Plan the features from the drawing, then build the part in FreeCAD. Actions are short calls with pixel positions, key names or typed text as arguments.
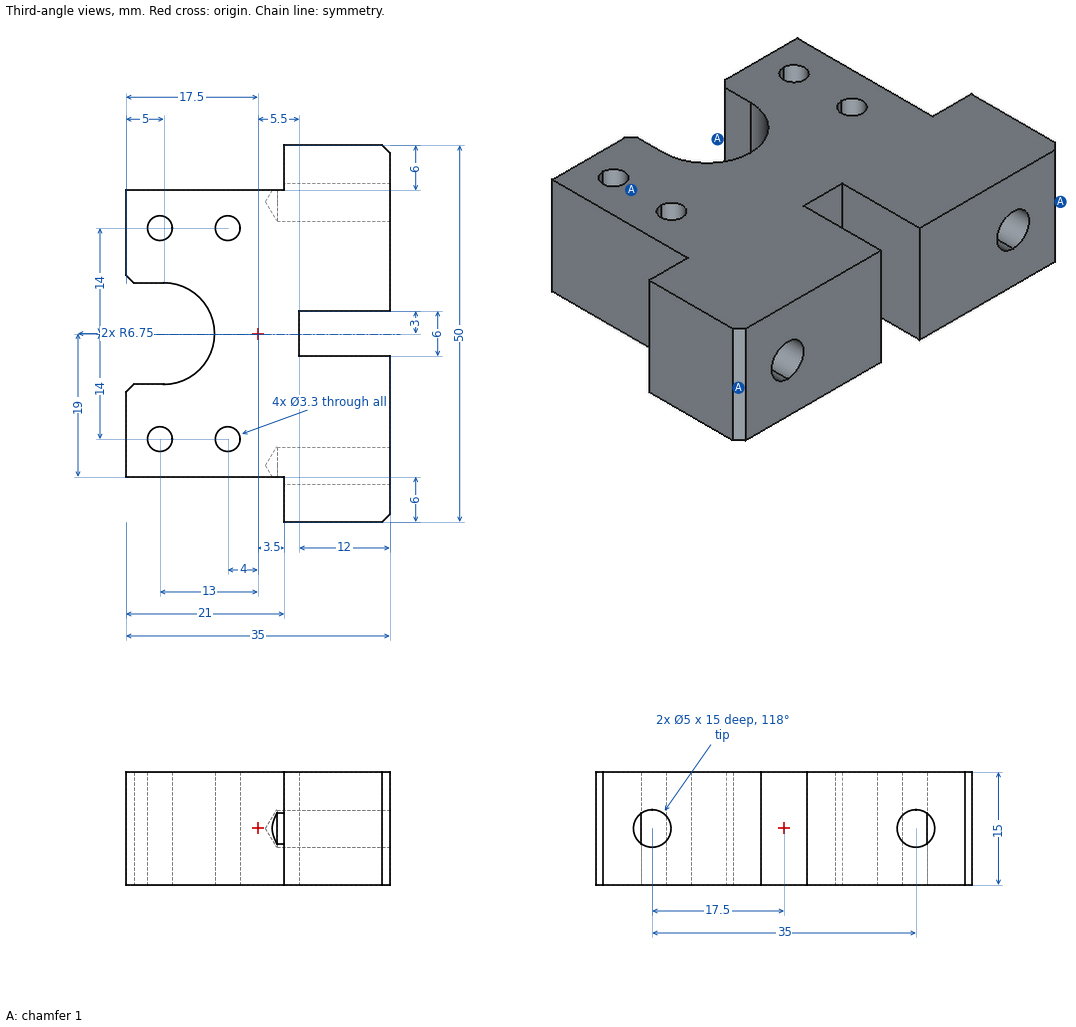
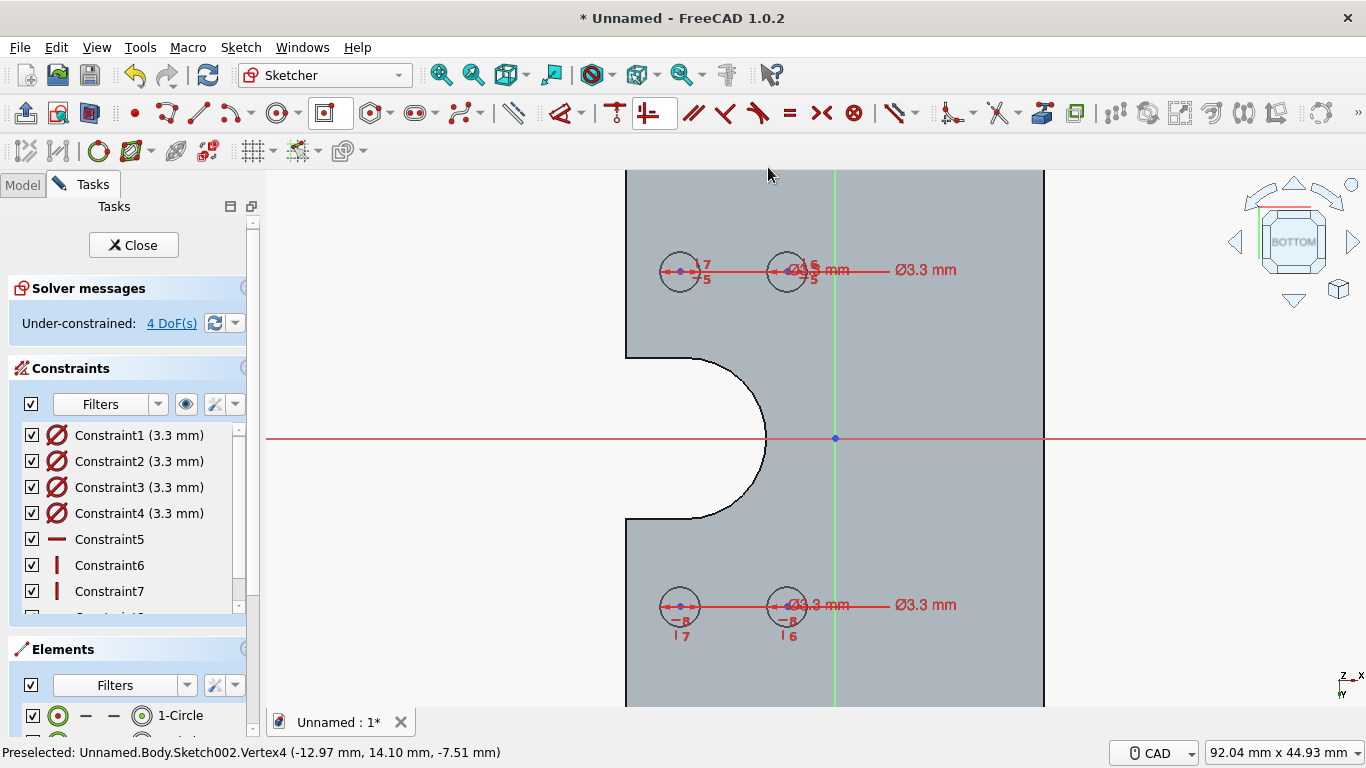
click(560, 114)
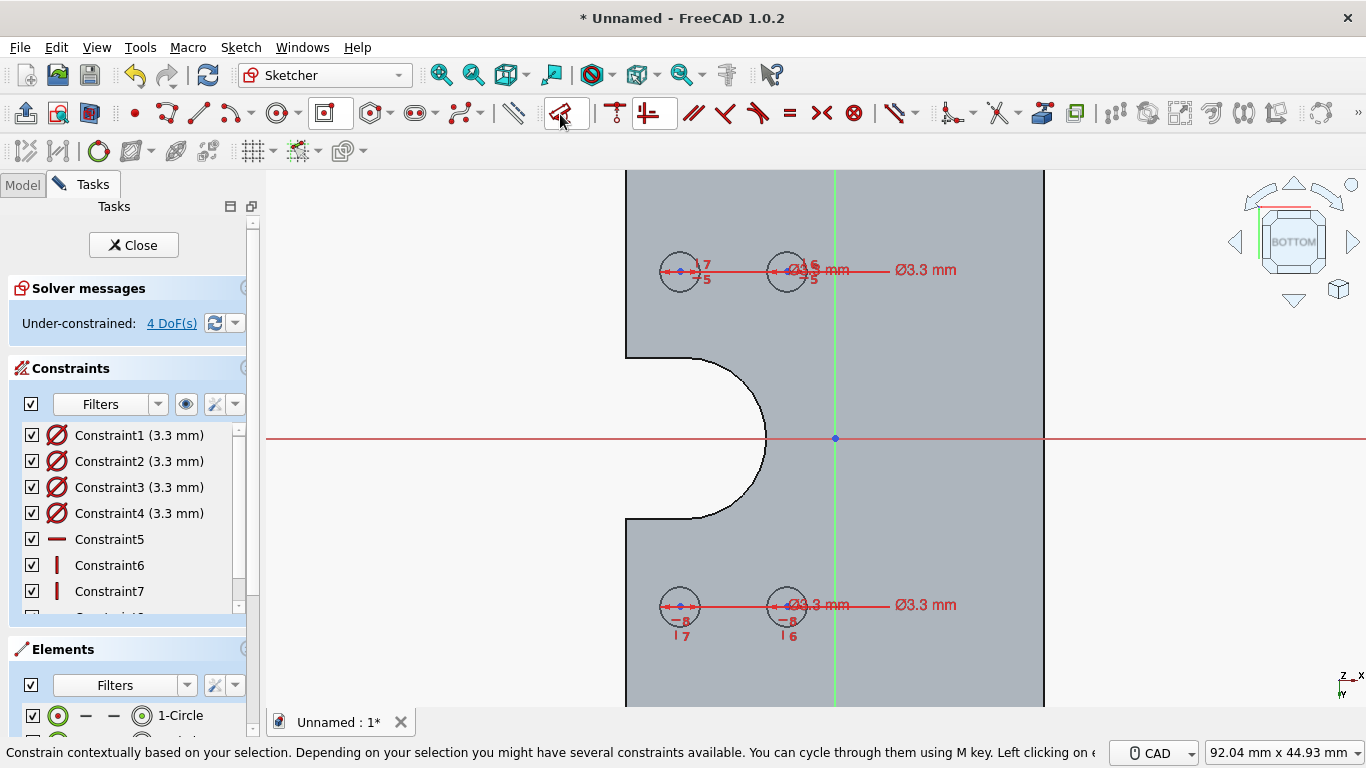
click(787, 272)
click(811, 238)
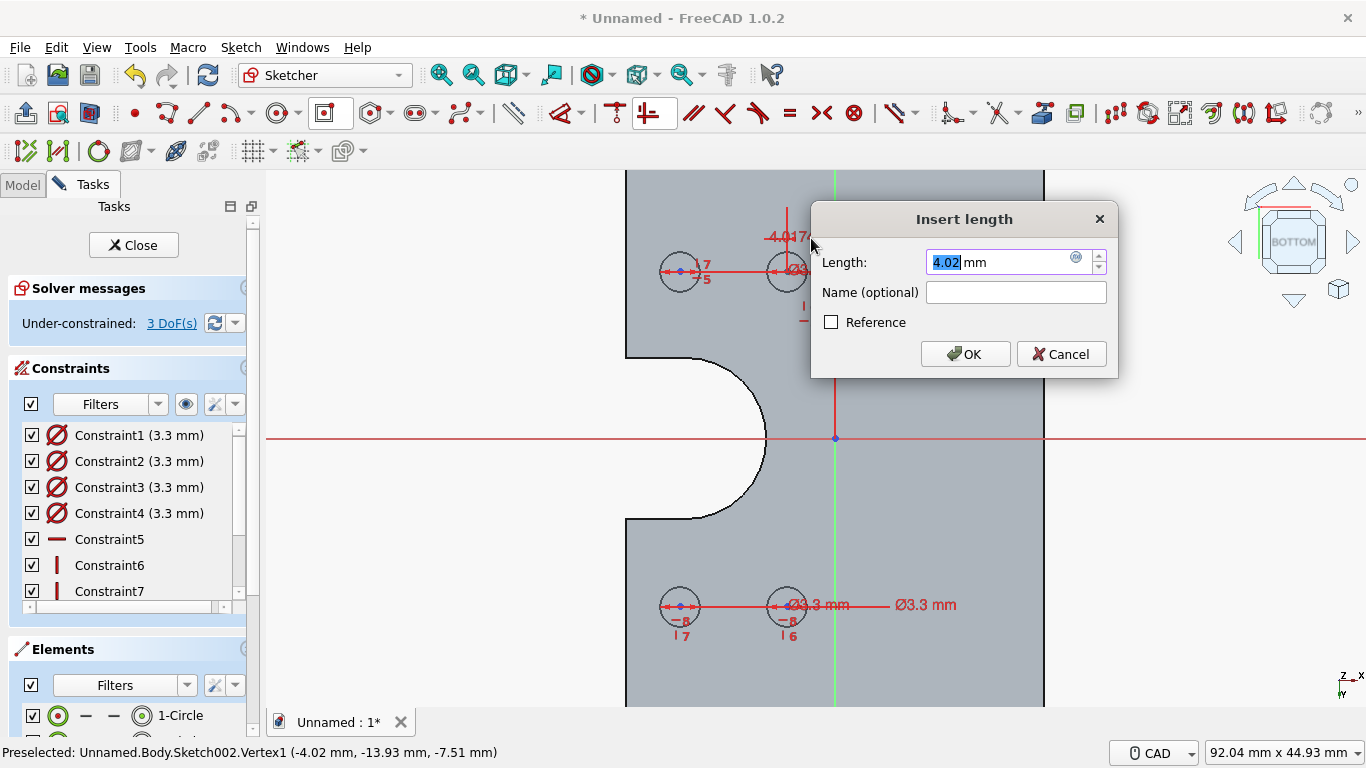
text(4)
key(Return)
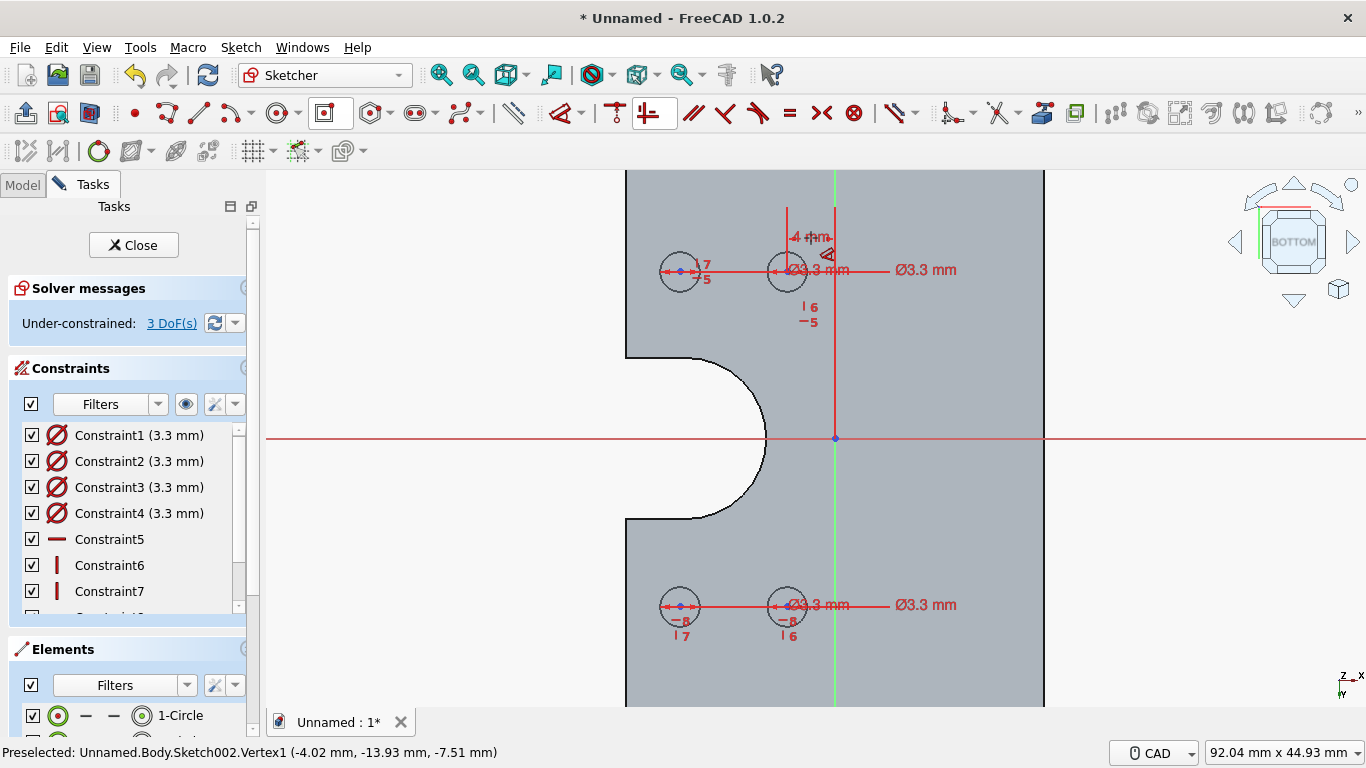
click(787, 272)
click(869, 355)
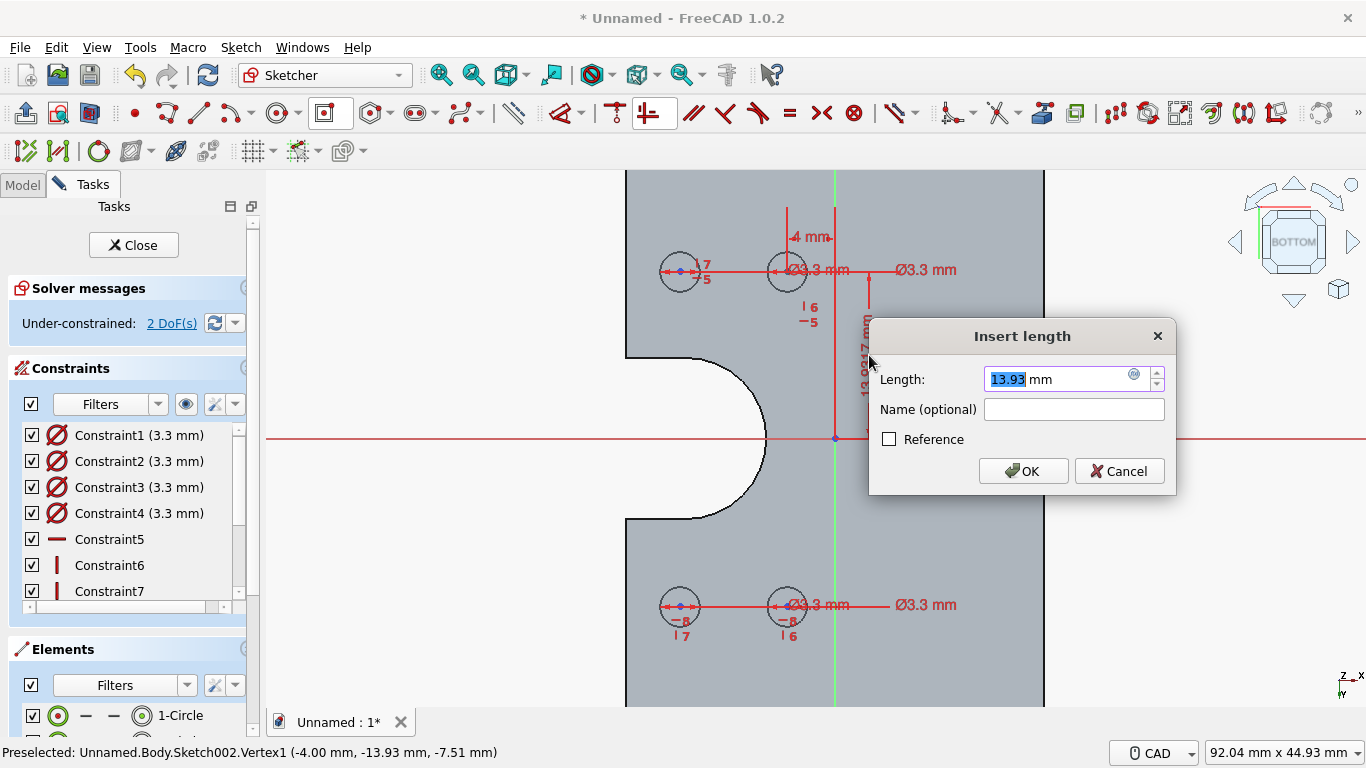
text(14)
key(Return)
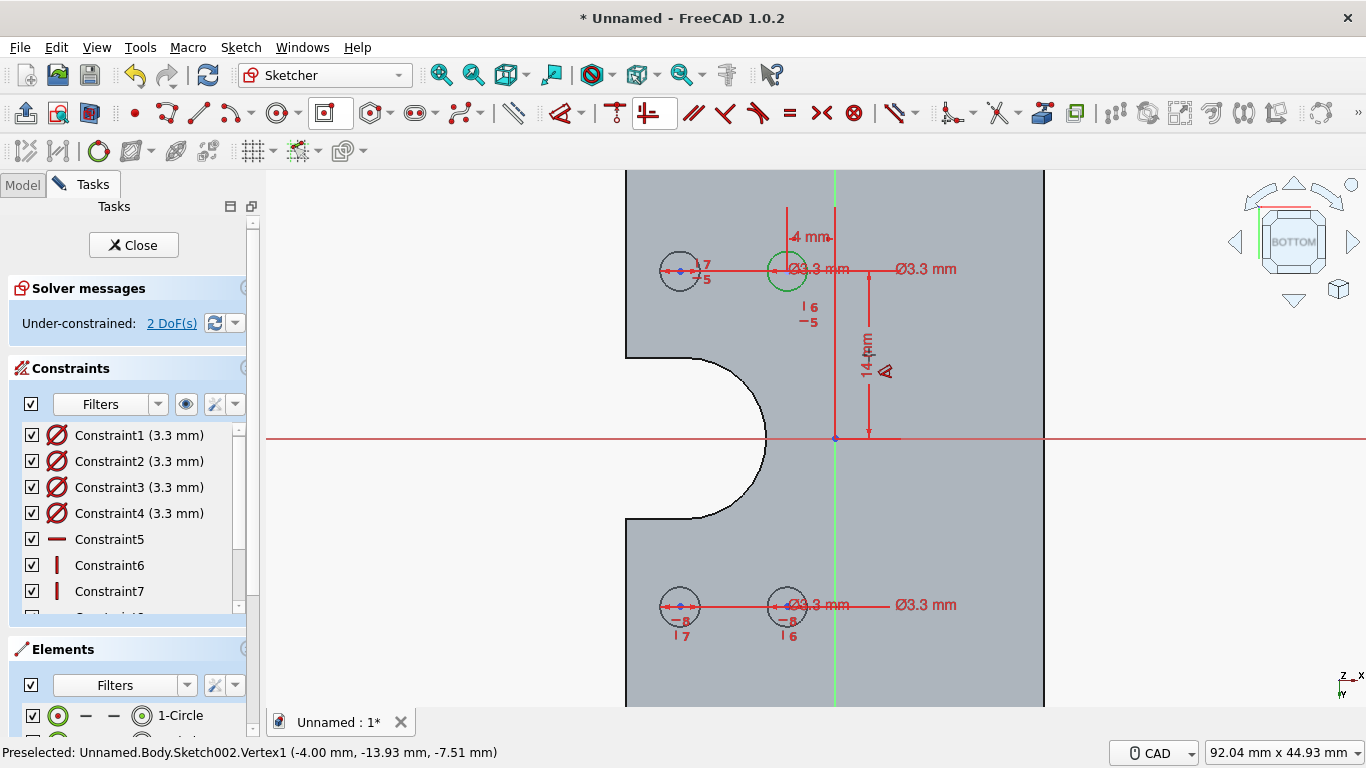
click(680, 271)
click(722, 237)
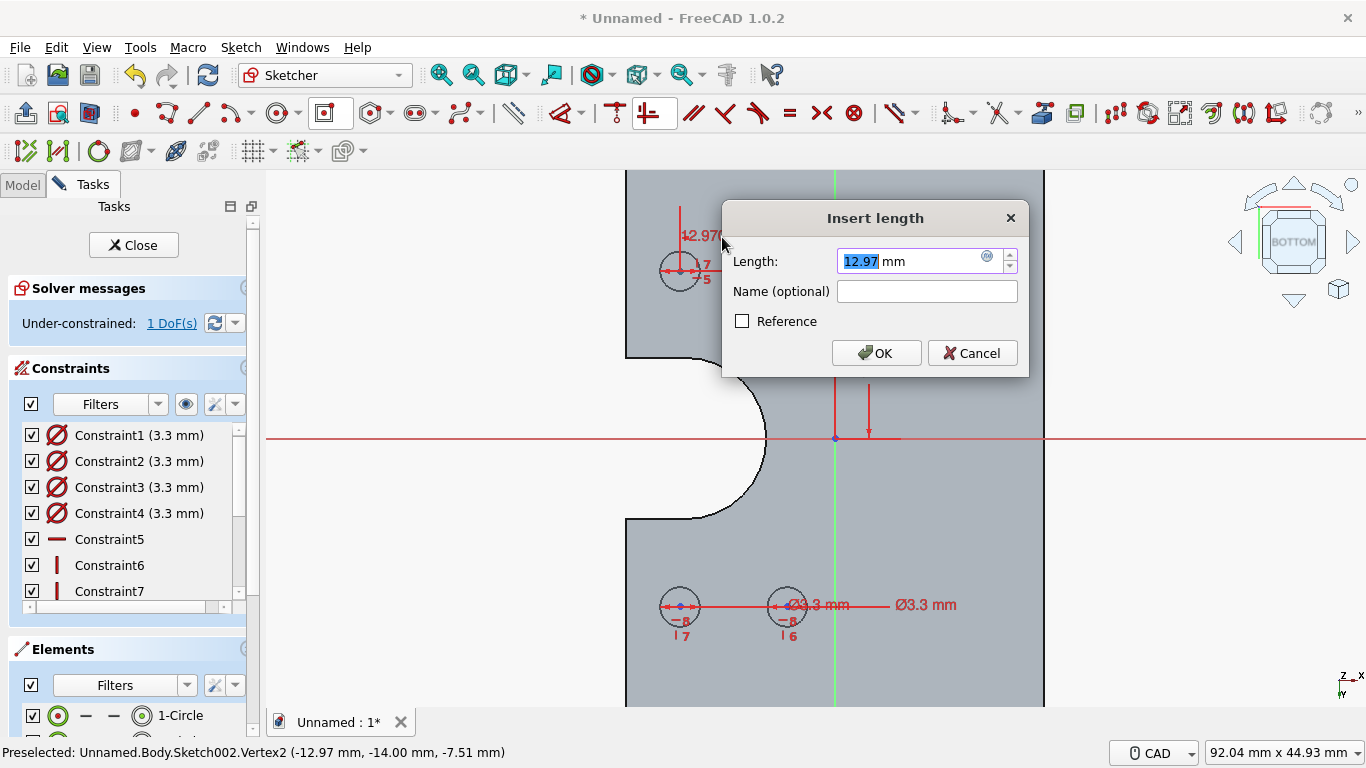
text(13)
key(Return)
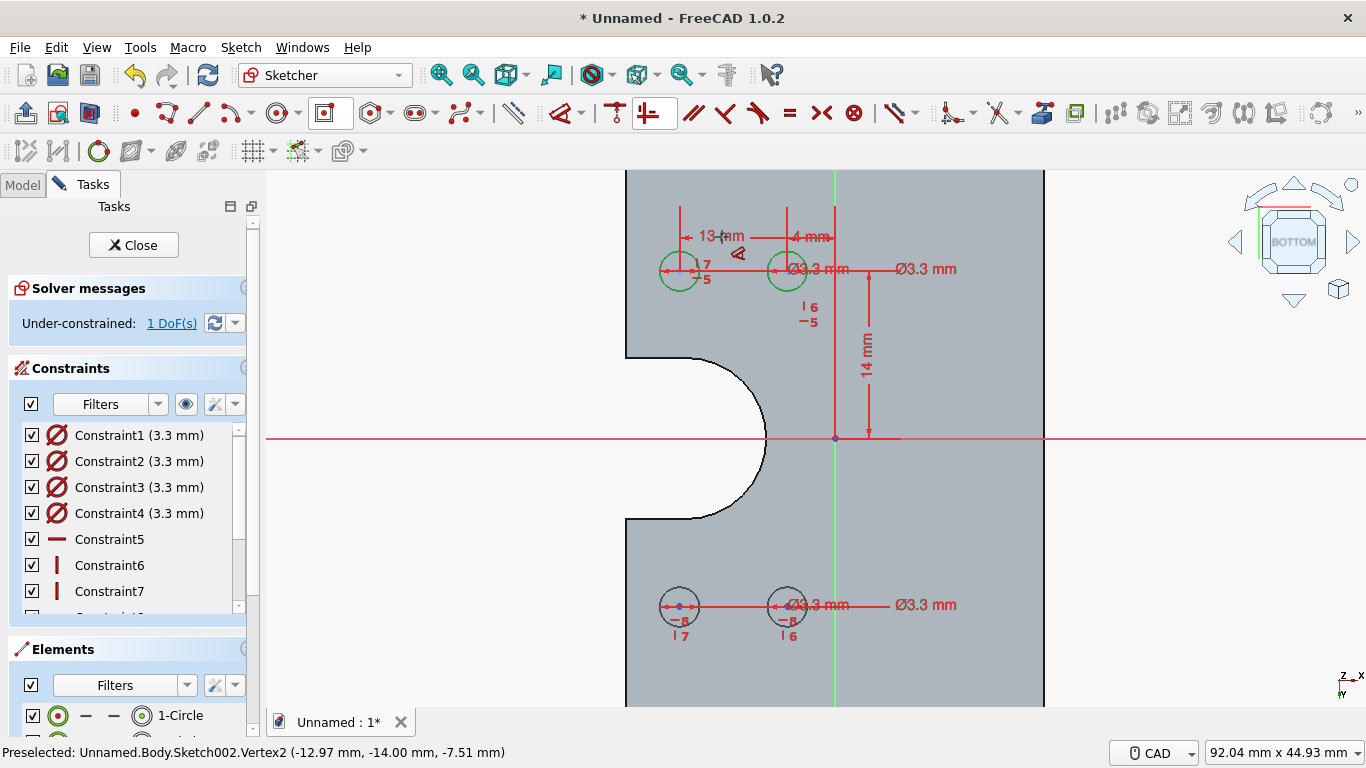
click(787, 607)
click(869, 523)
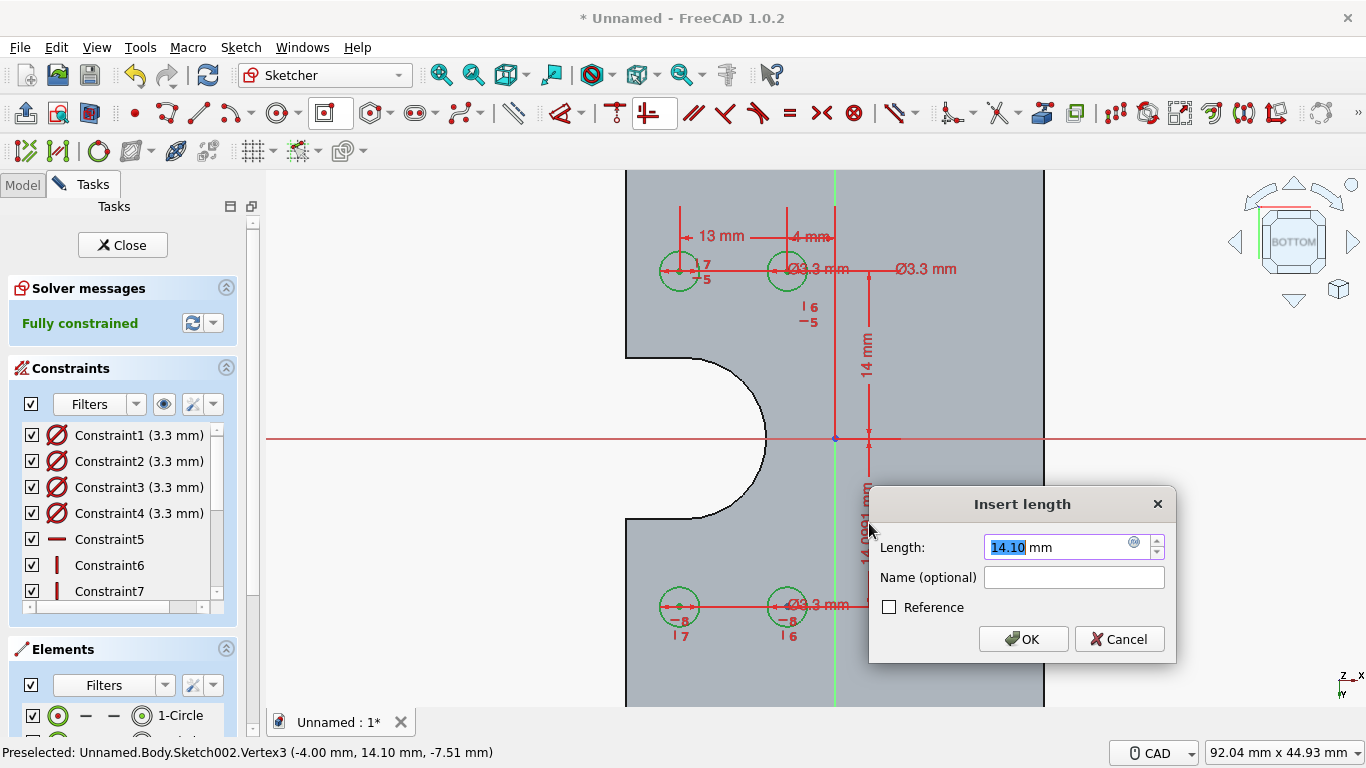
text(14)
key(Return)
key(Escape)